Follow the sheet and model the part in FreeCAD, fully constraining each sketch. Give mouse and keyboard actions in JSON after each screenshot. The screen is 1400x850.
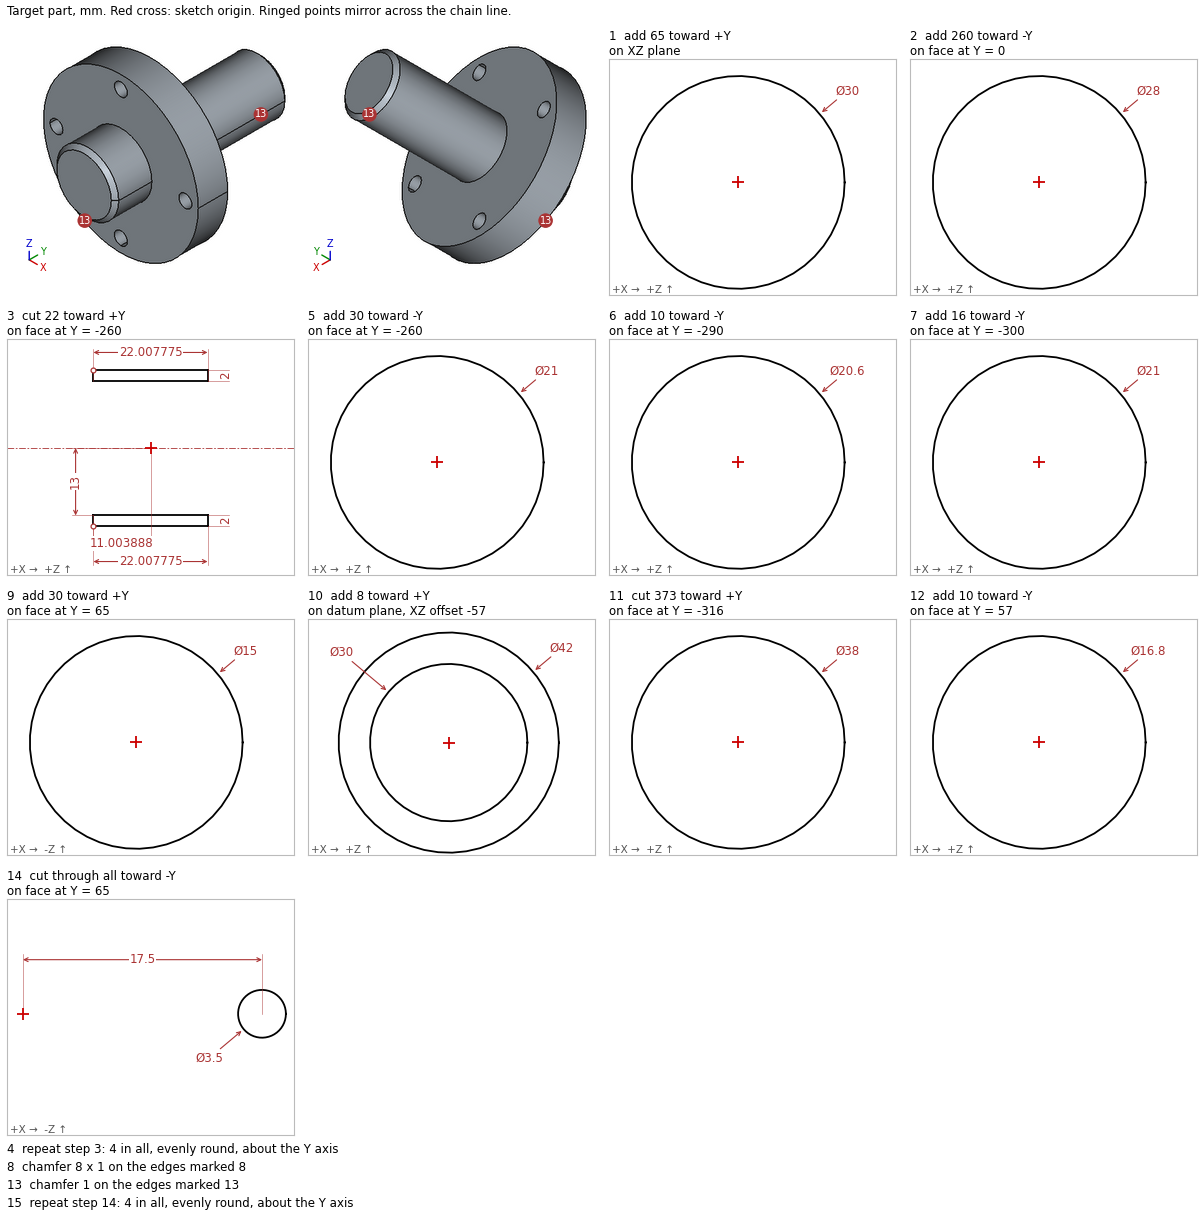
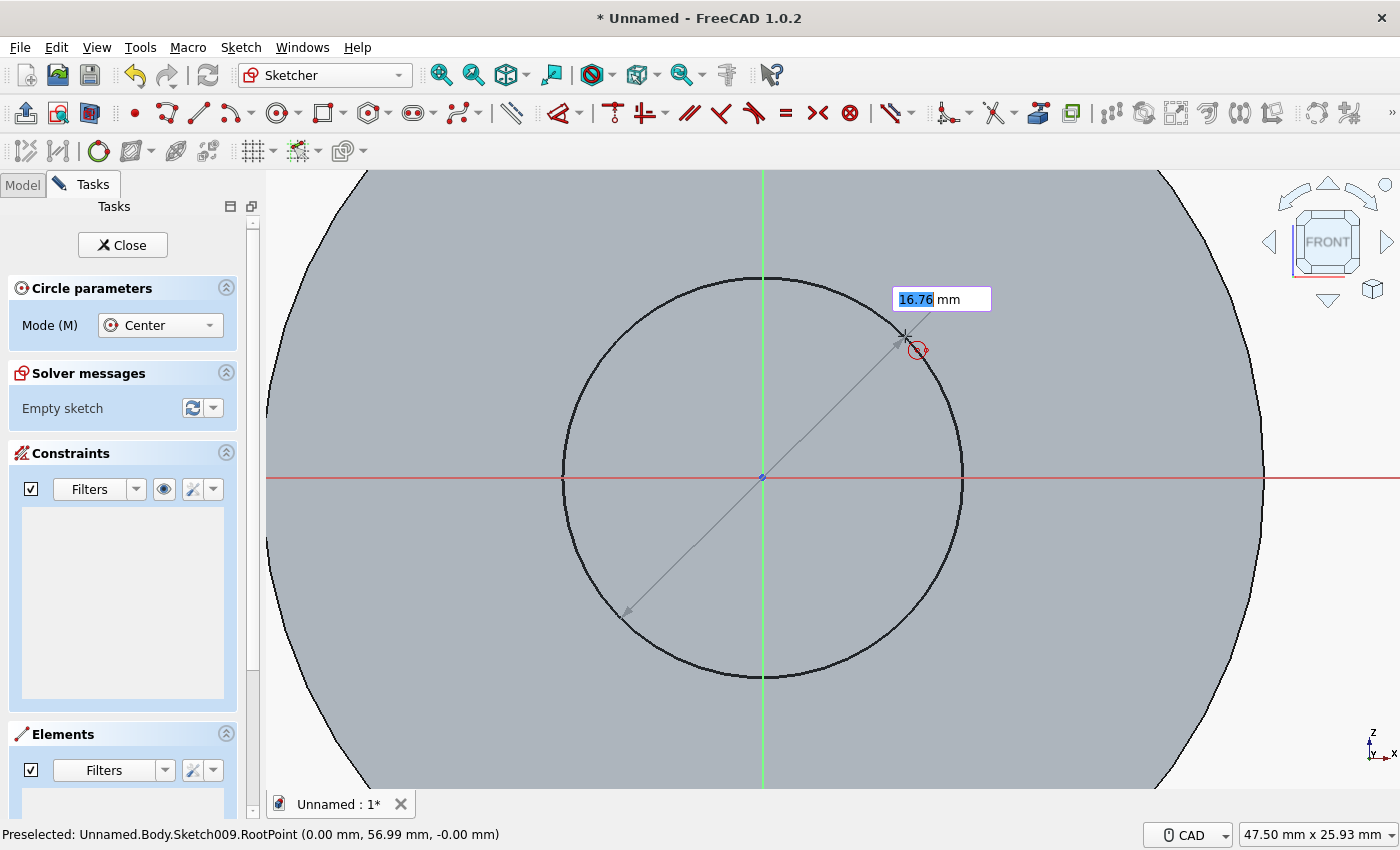
{"action": "type", "text": "16.8"}
{"action": "key", "text": "Return"}
{"action": "key", "text": "Escape"}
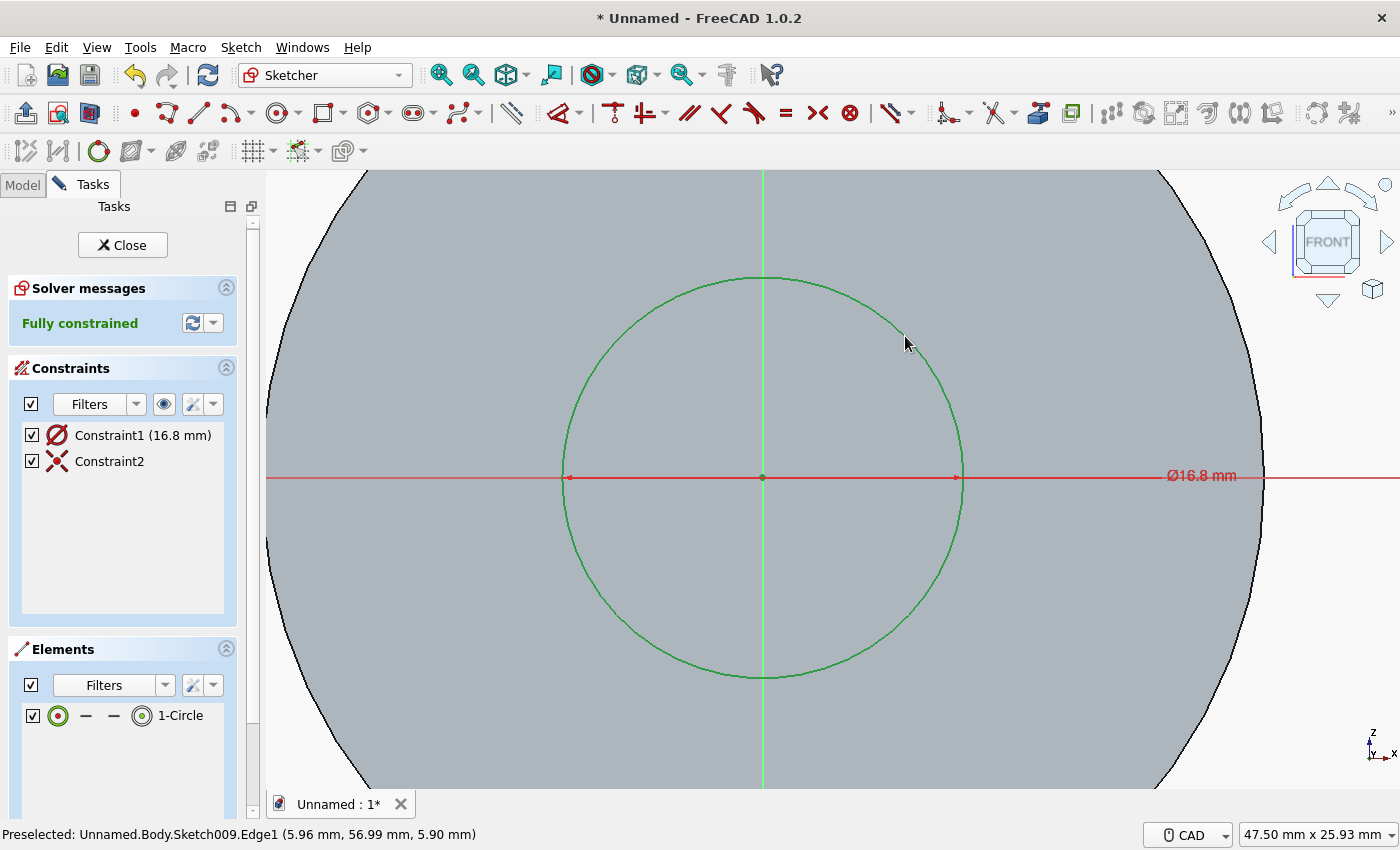
{"action": "left_click", "coordinate": [123, 245]}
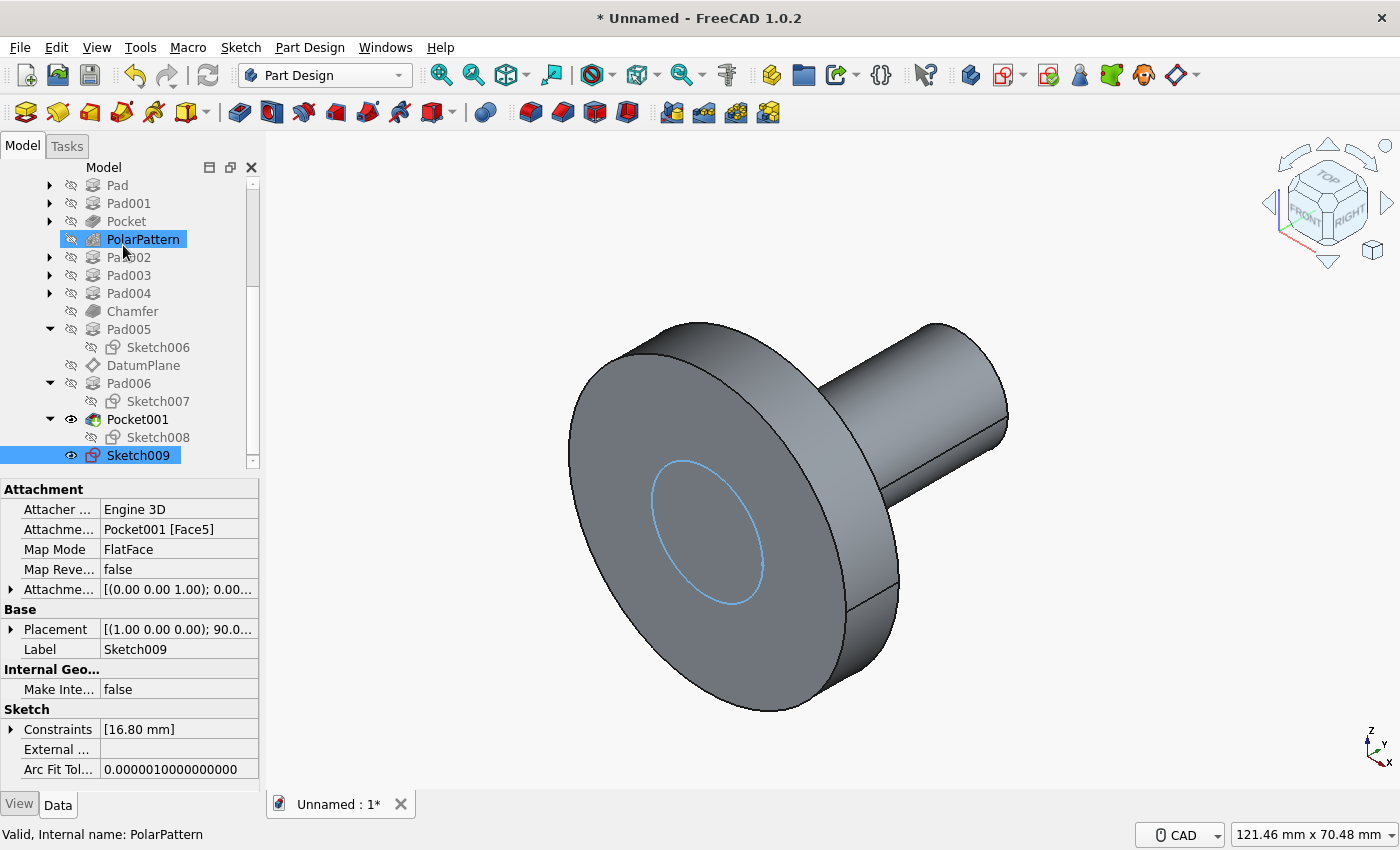
{"action": "left_click", "coordinate": [26, 112]}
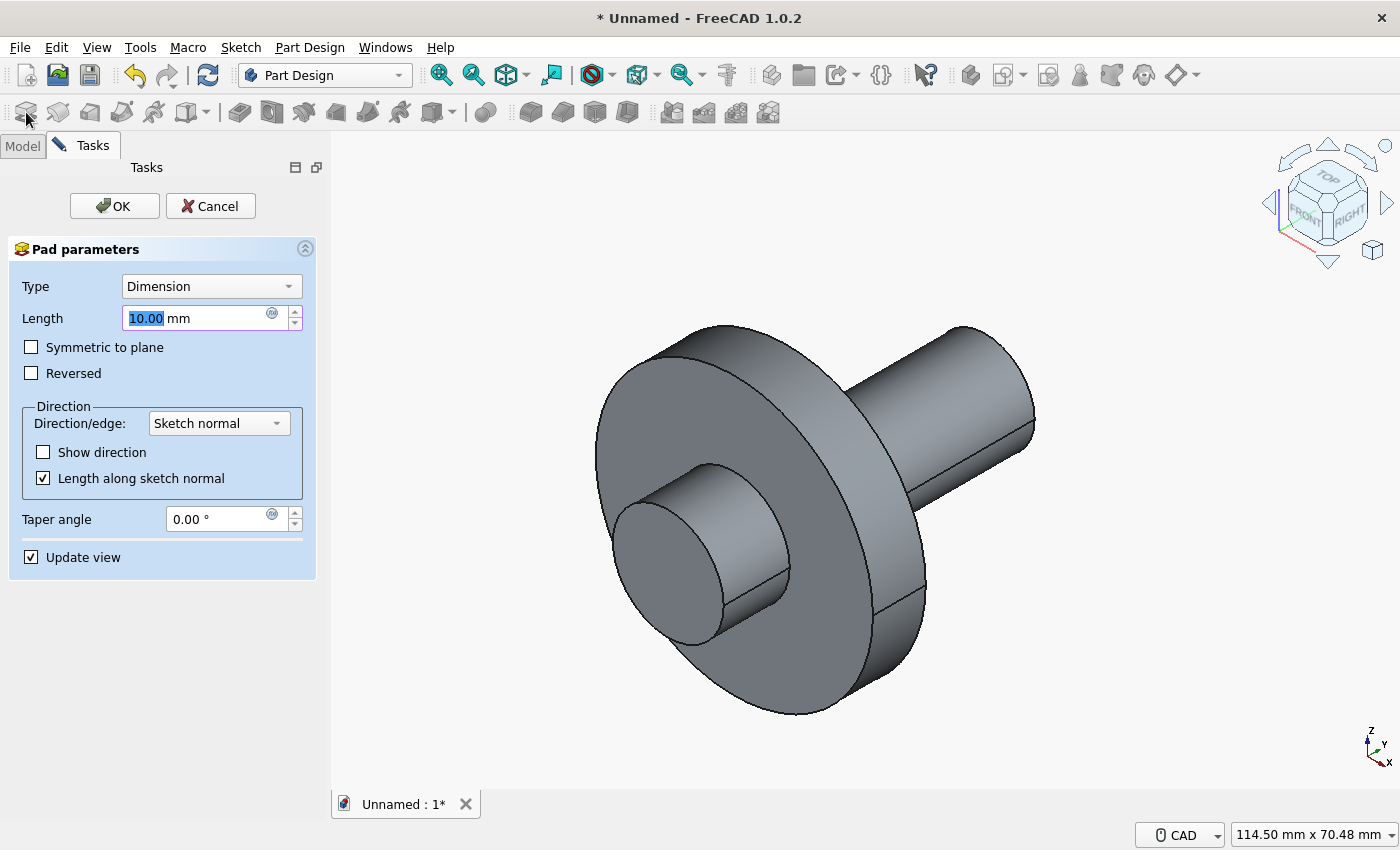
{"action": "type", "text": "10"}
{"action": "key", "text": "Tab"}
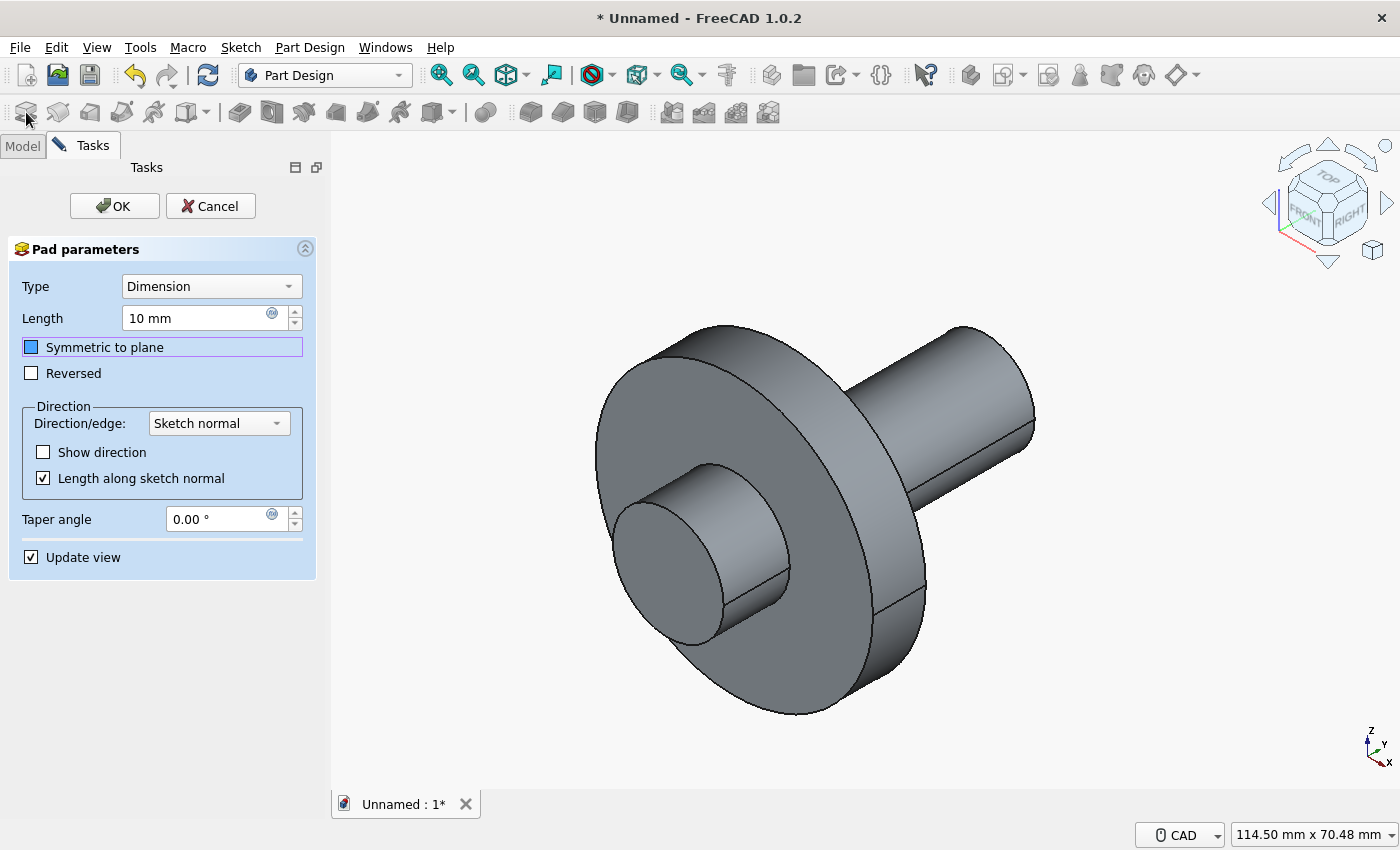
{"action": "left_click", "coordinate": [115, 206]}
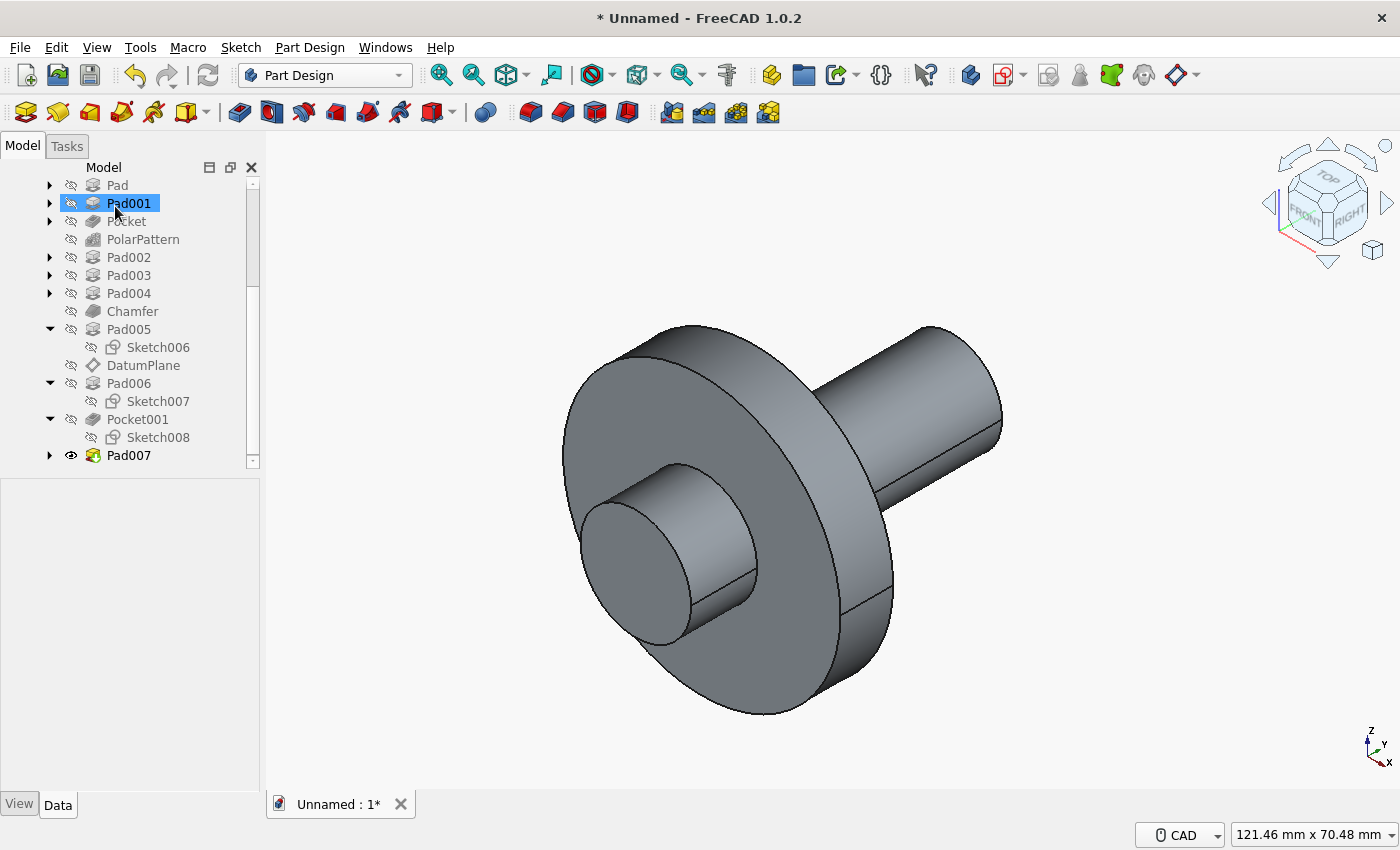
{"action": "left_click", "coordinate": [442, 76]}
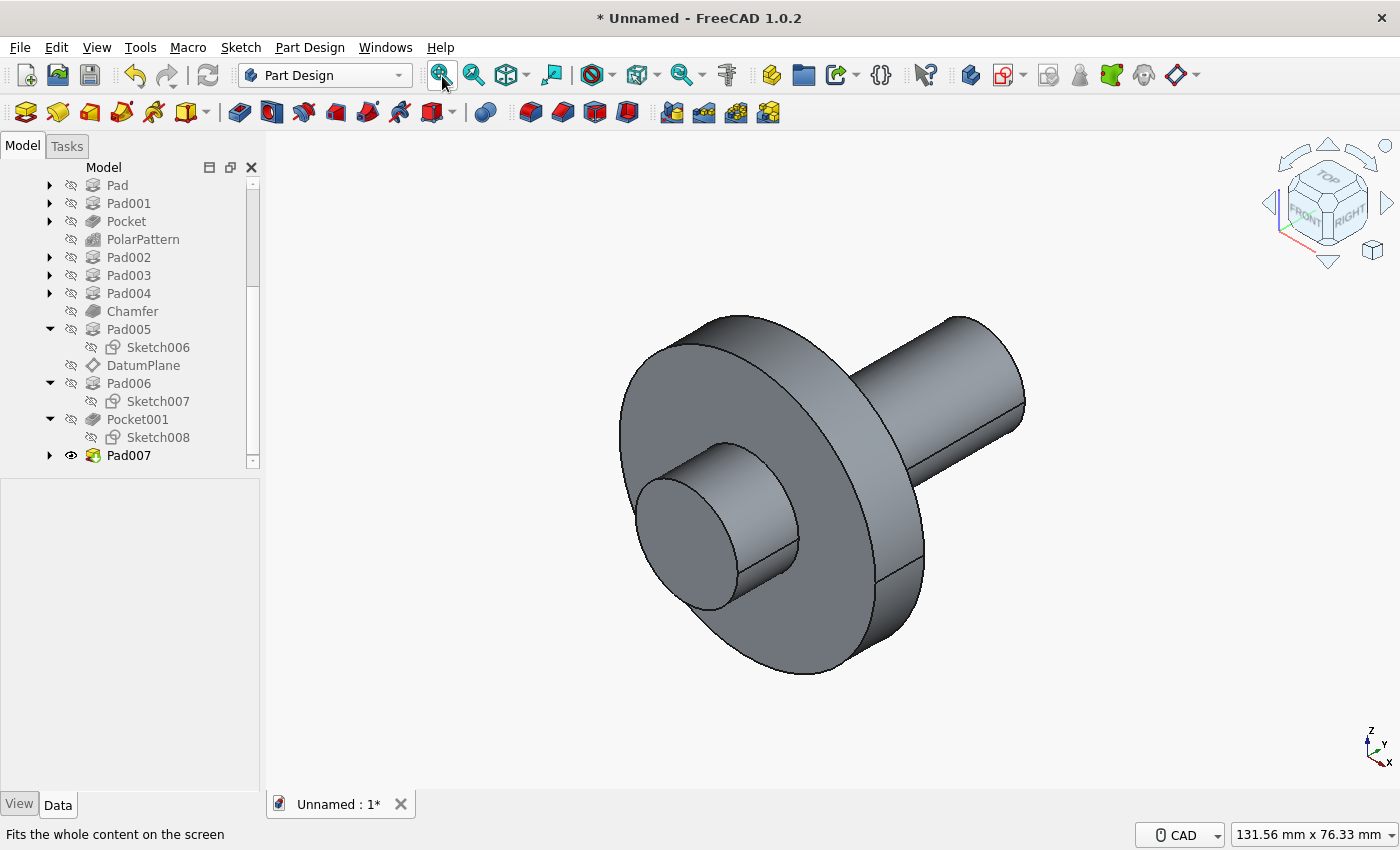
{"action": "left_click", "coordinate": [965, 316]}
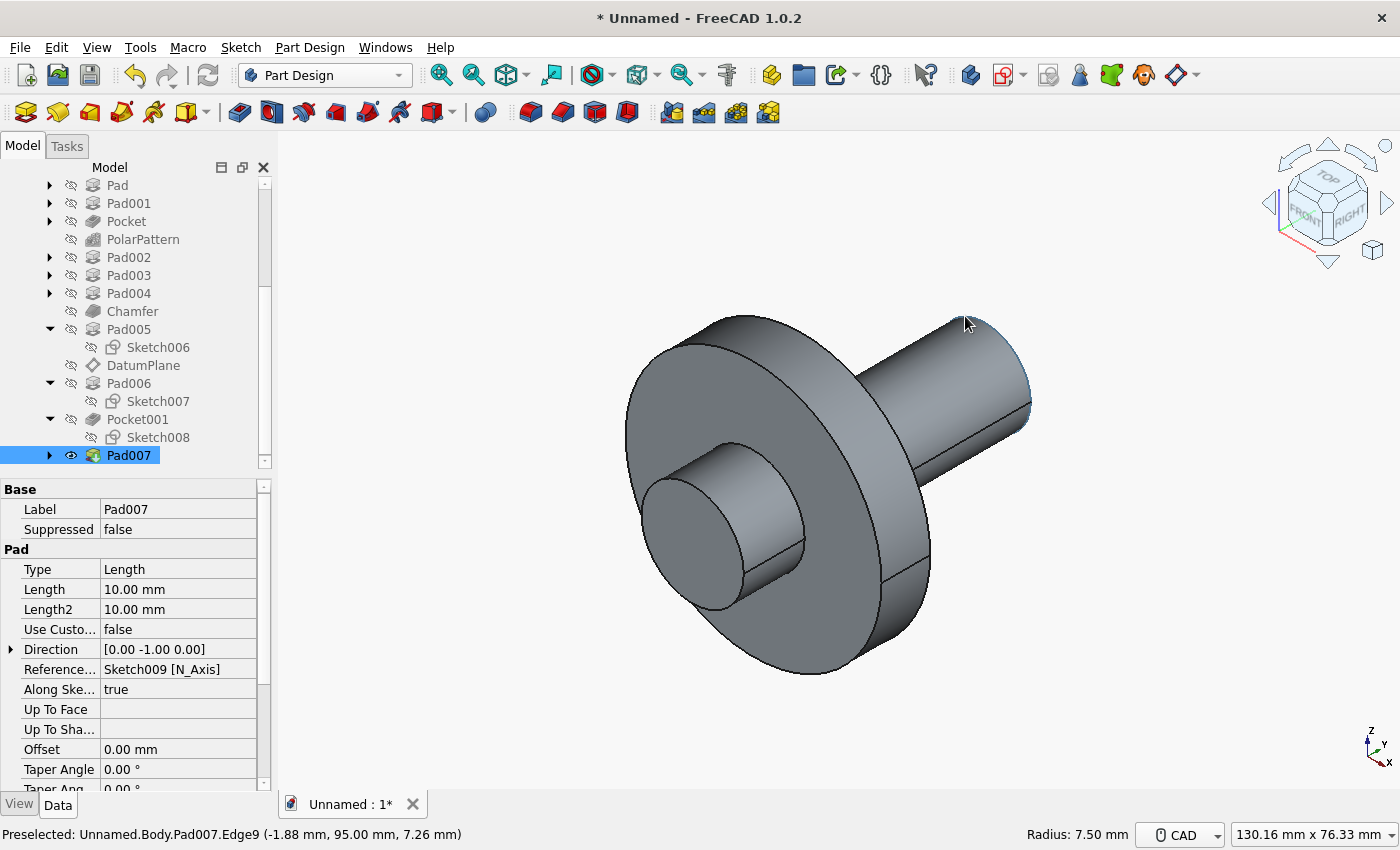
{"action": "left_click", "coordinate": [677, 478], "text": "ctrl"}